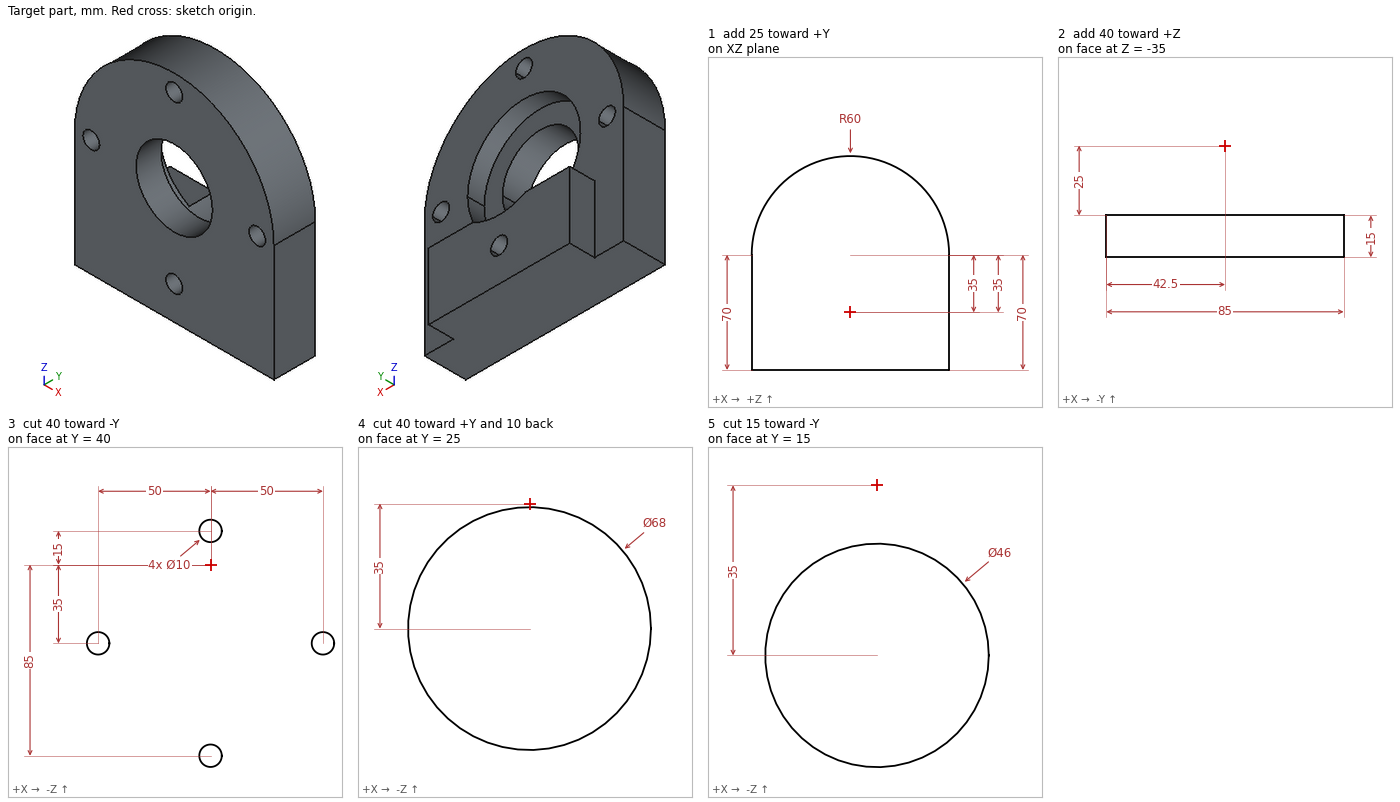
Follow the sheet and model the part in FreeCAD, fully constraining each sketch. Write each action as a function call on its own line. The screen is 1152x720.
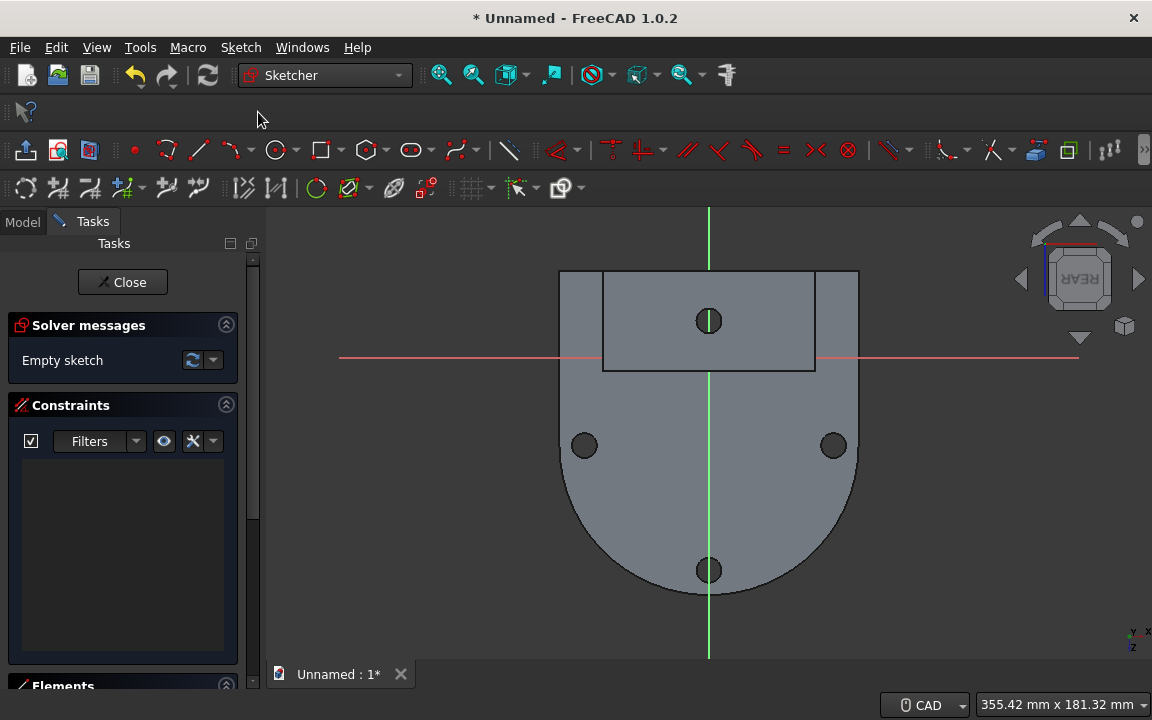
click(90, 150)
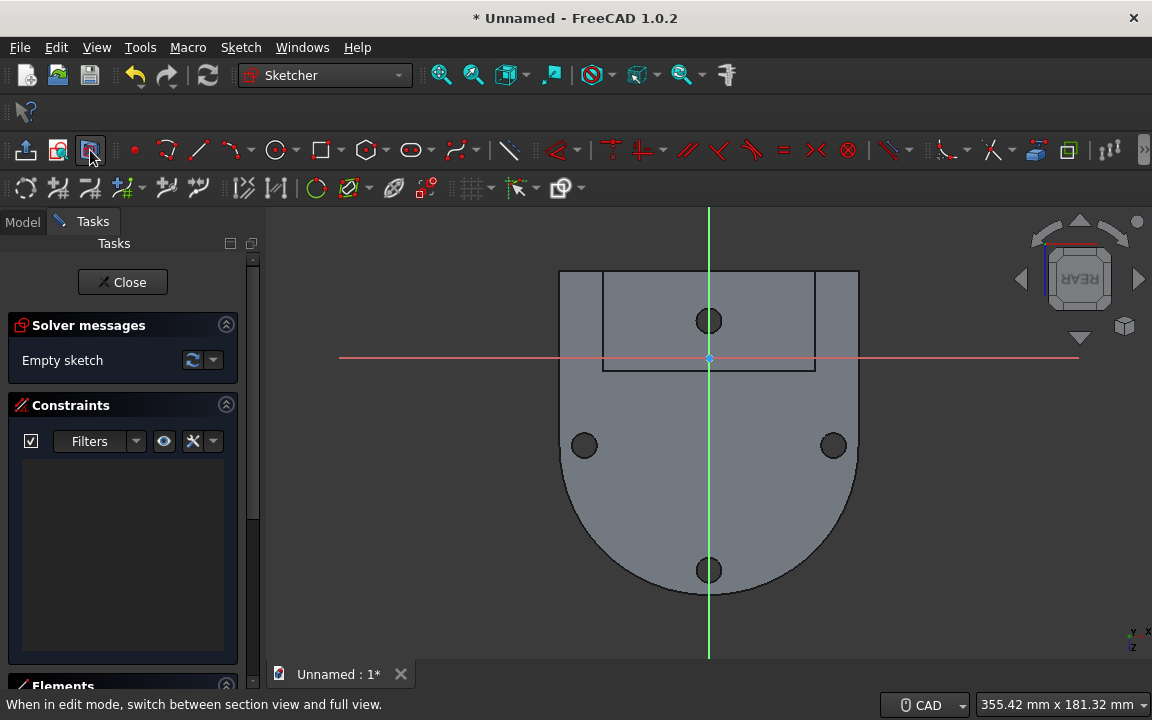
scroll(848, 467, up, 2)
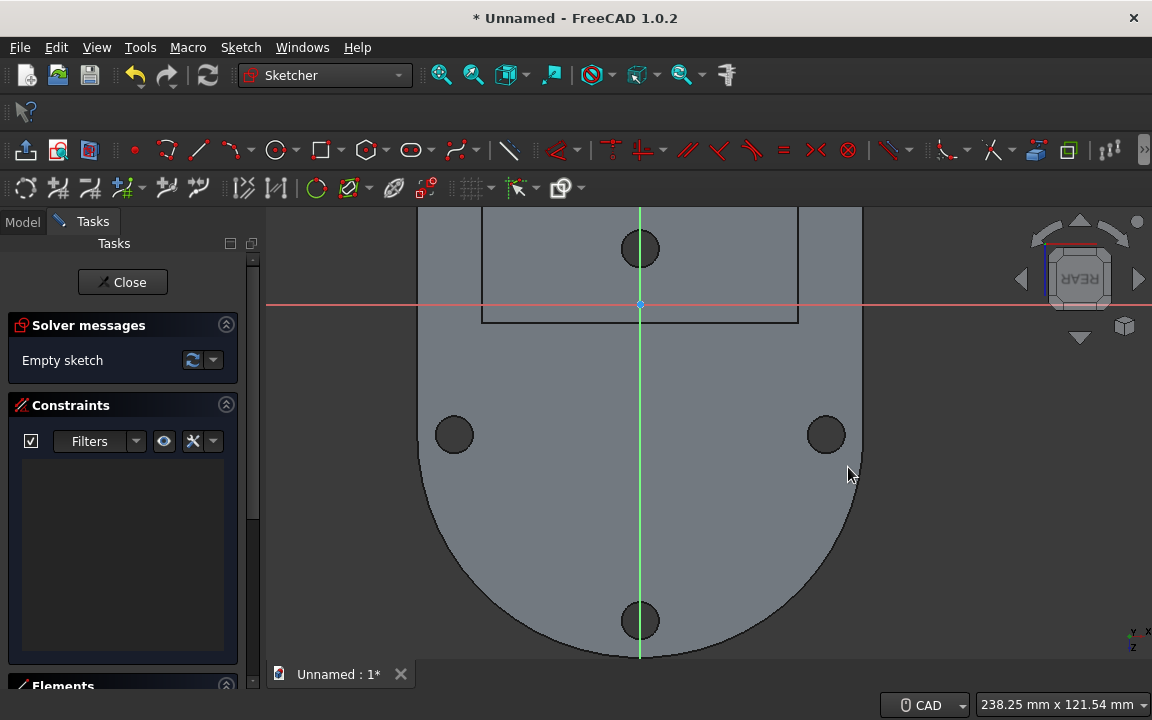
key(g)
key(c)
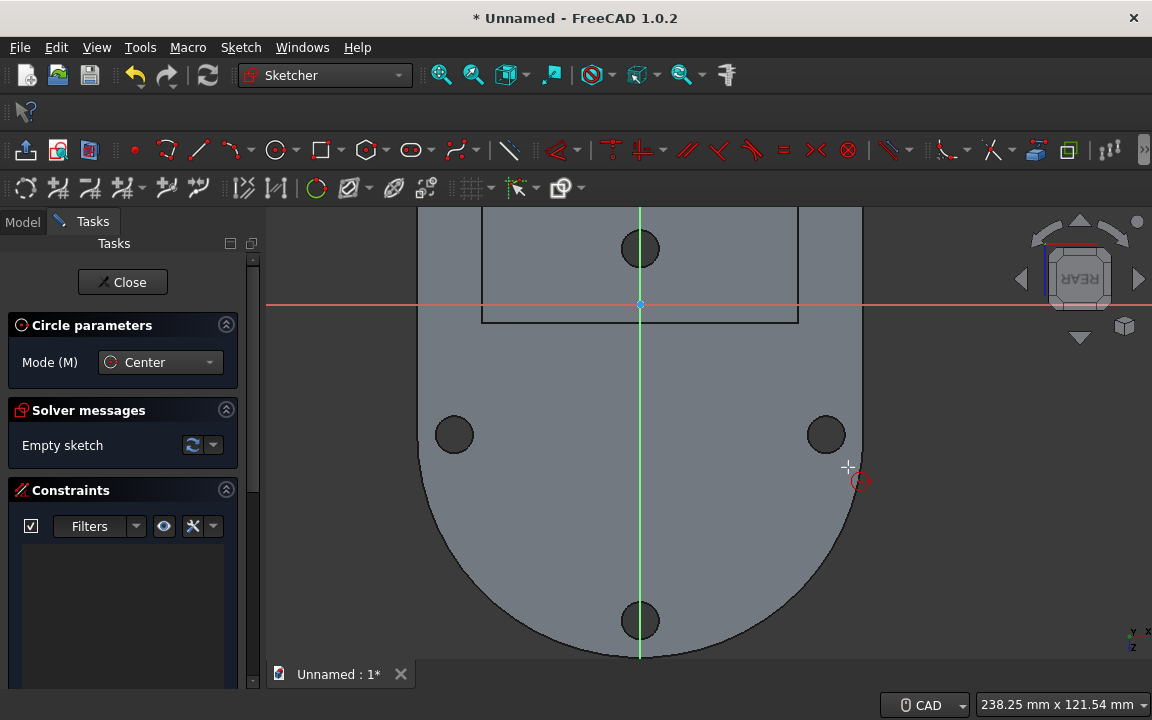
click(640, 435)
move(730, 345)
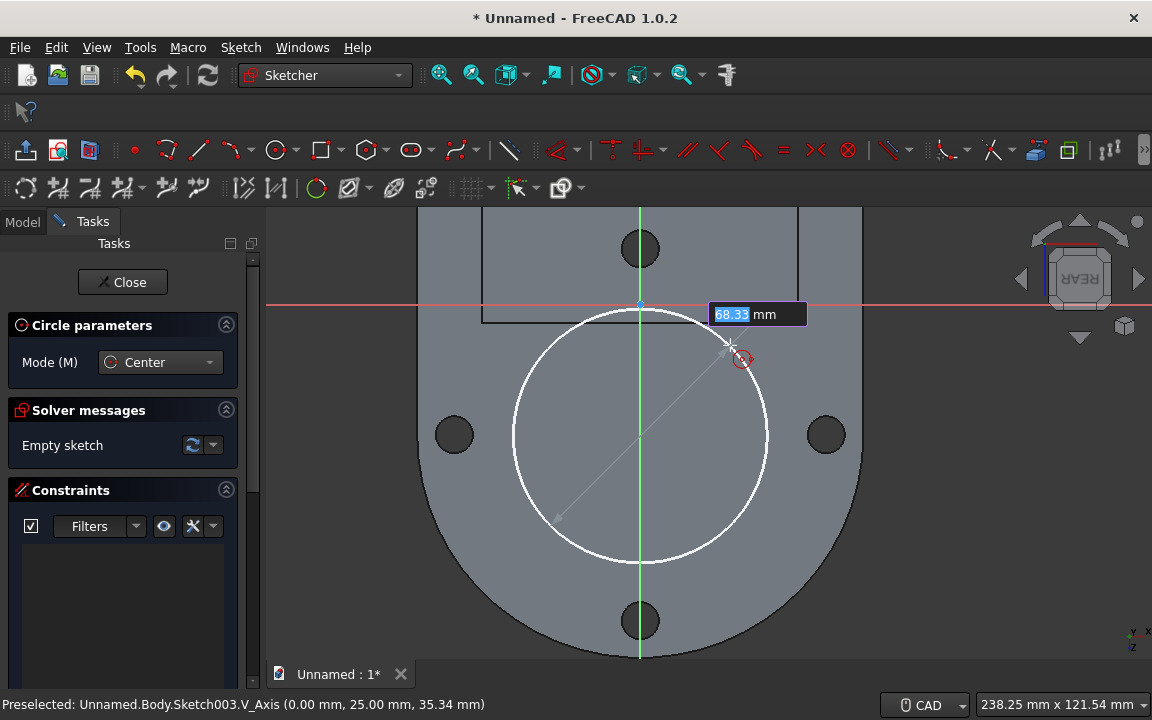
text(68)
key(Return)
key(Escape)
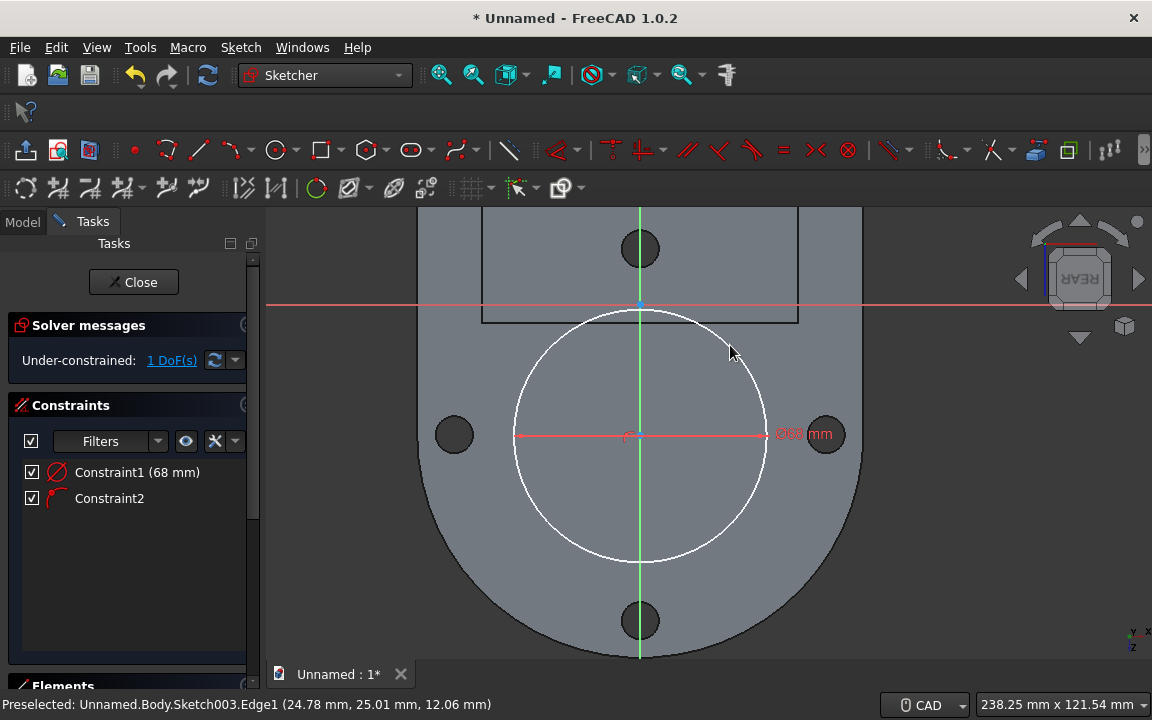
key(d)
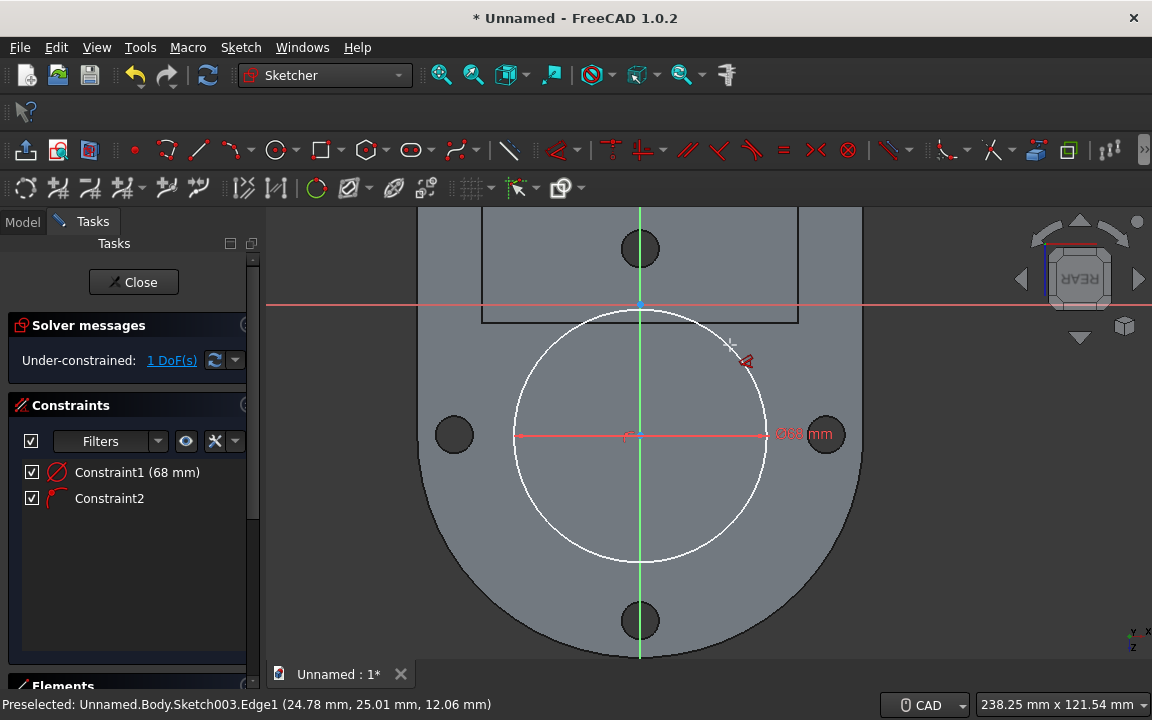
click(640, 436)
click(674, 370)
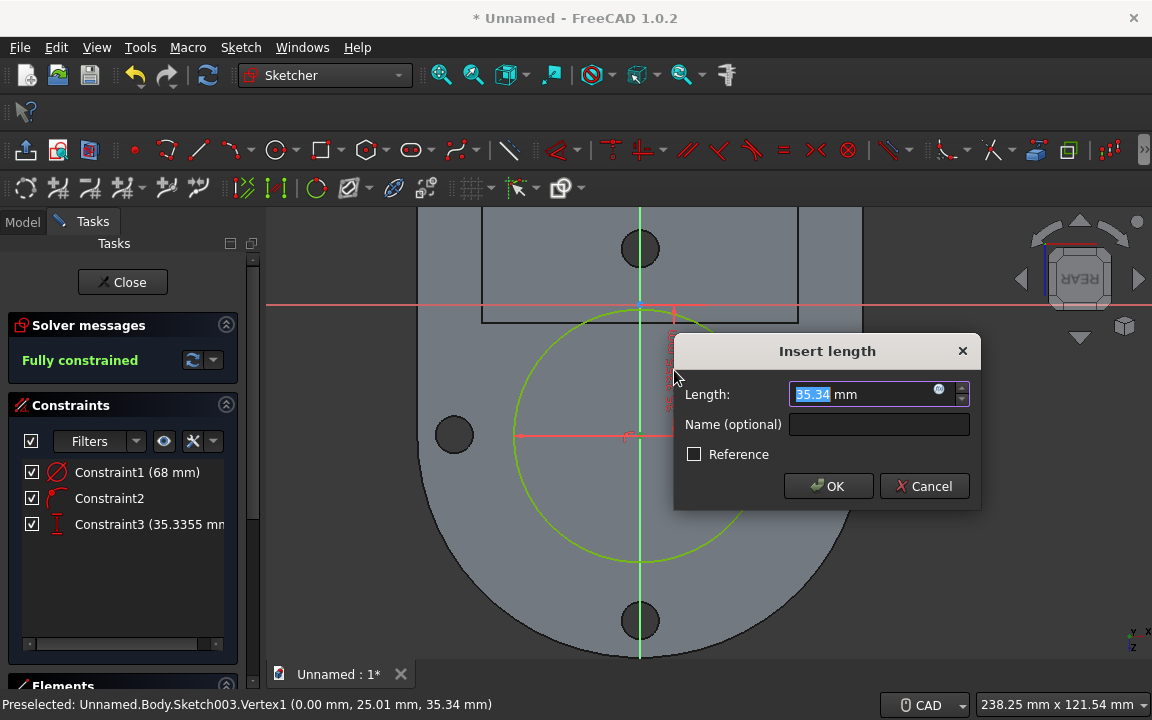
text(35)
key(Return)
key(Escape)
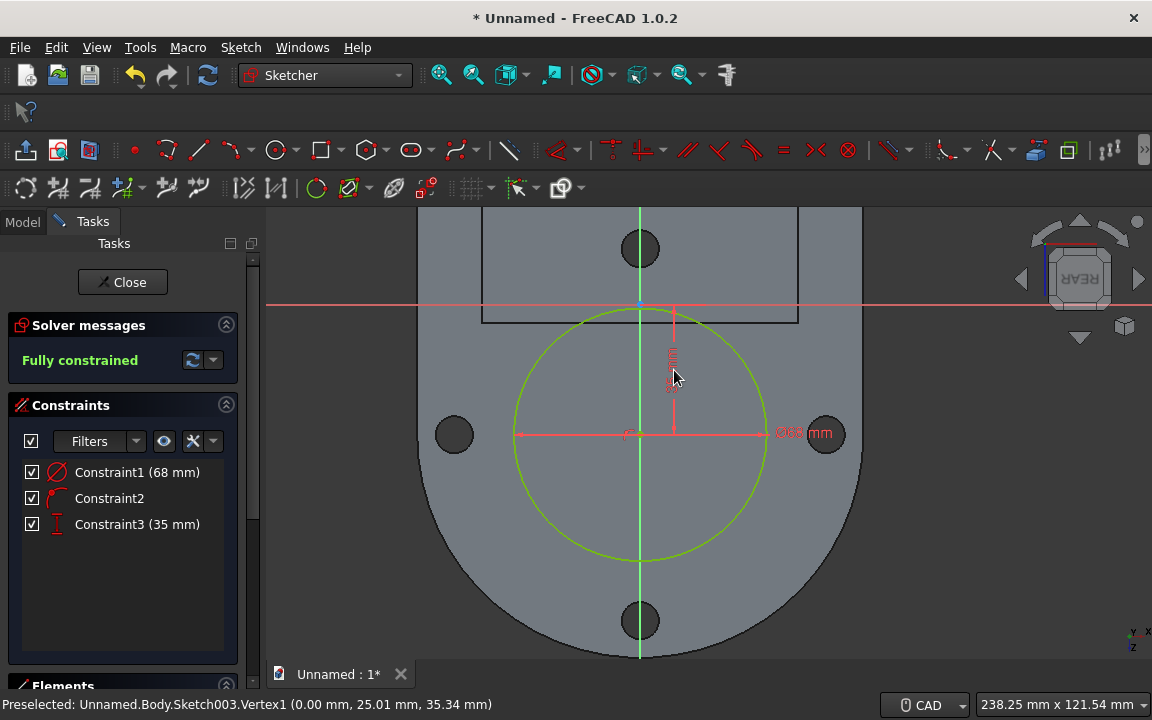
click(123, 282)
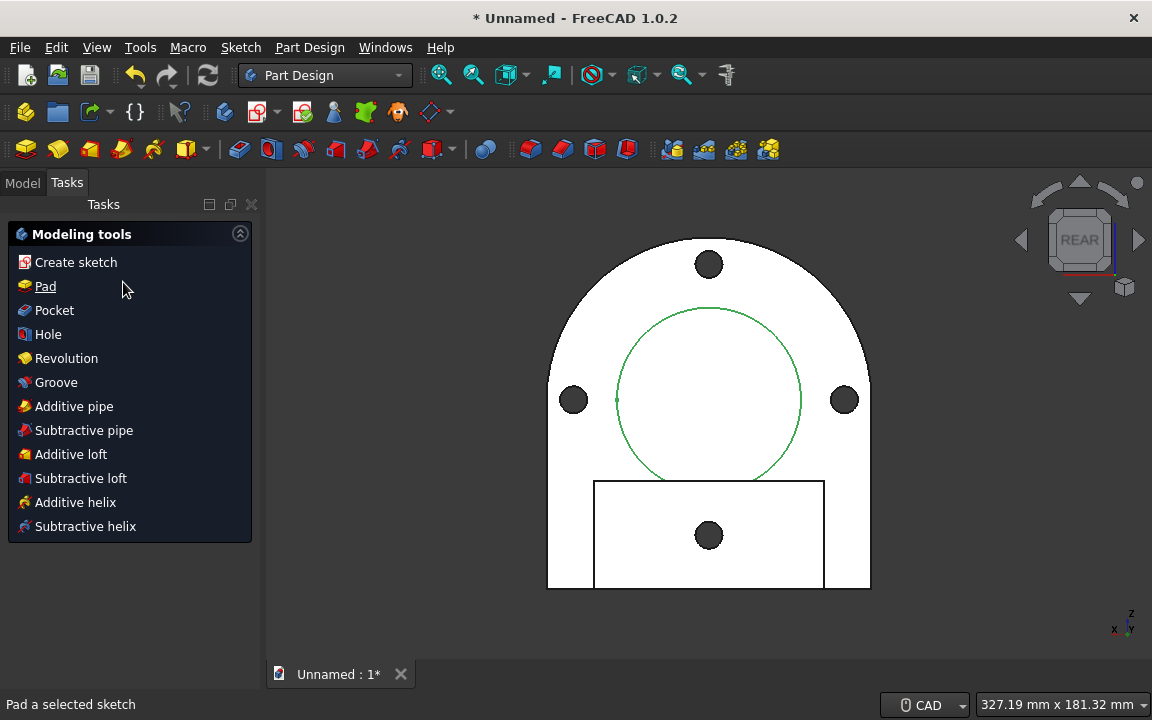
click(240, 150)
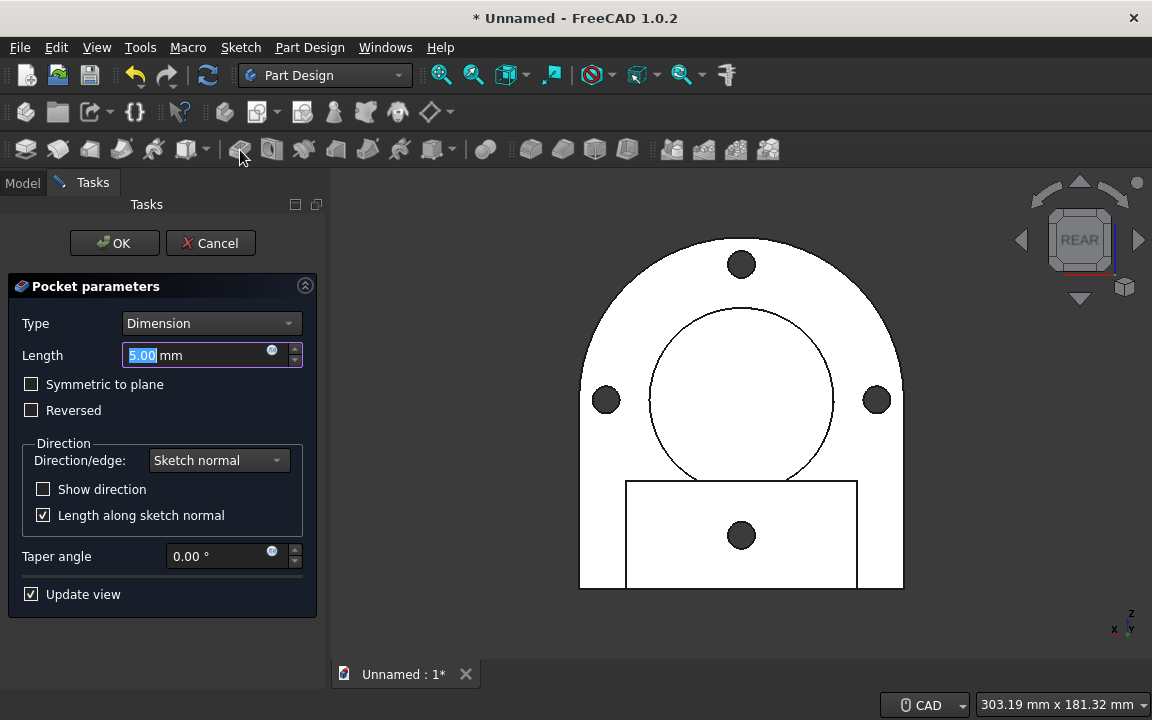
click(212, 324)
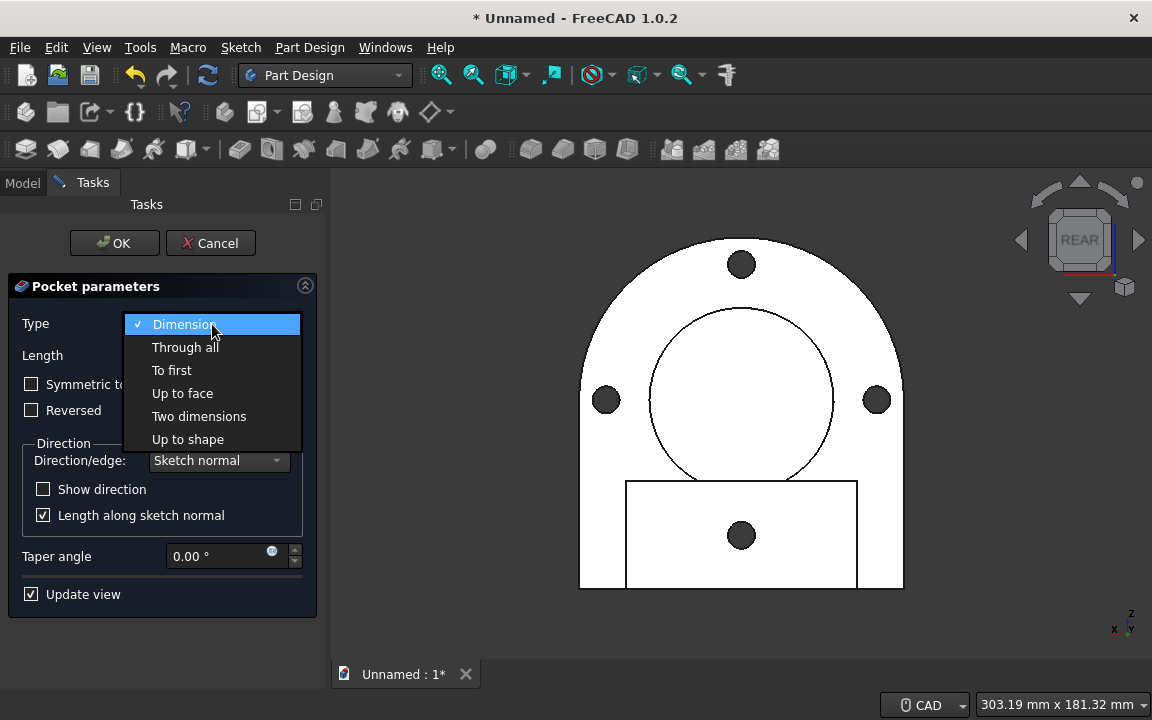
click(212, 416)